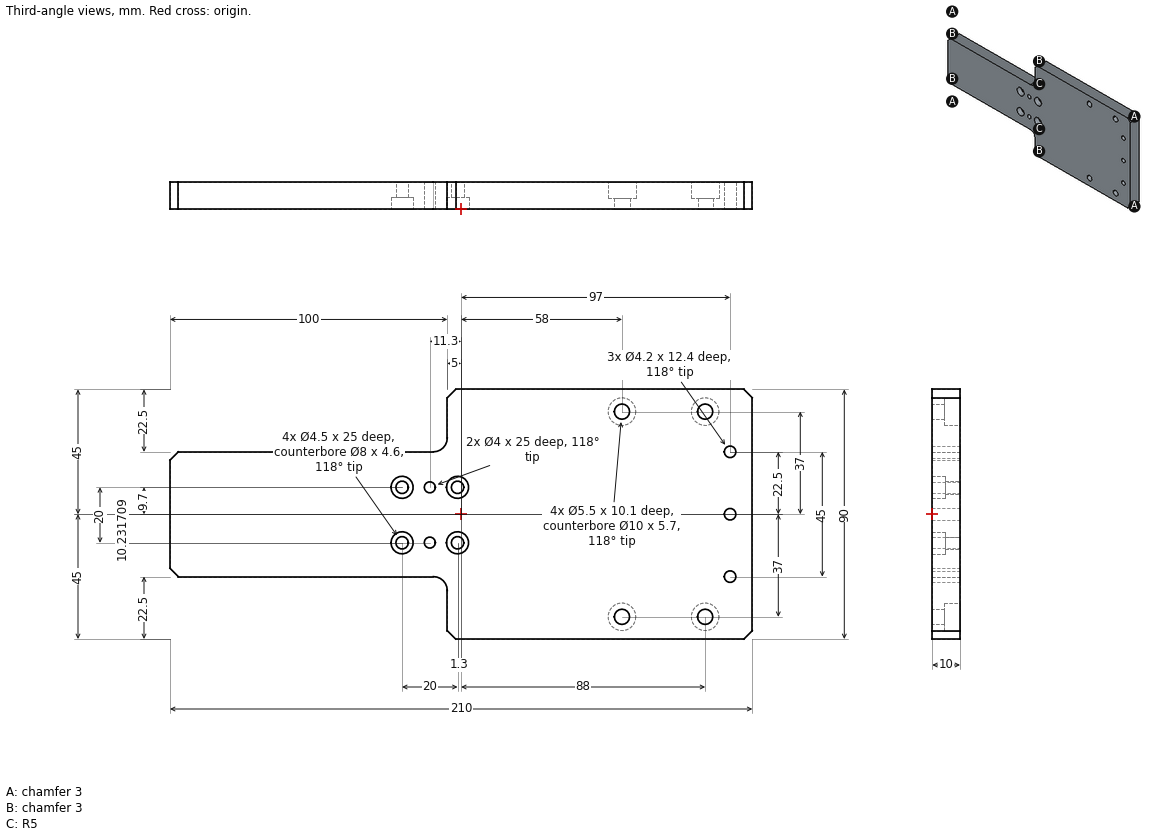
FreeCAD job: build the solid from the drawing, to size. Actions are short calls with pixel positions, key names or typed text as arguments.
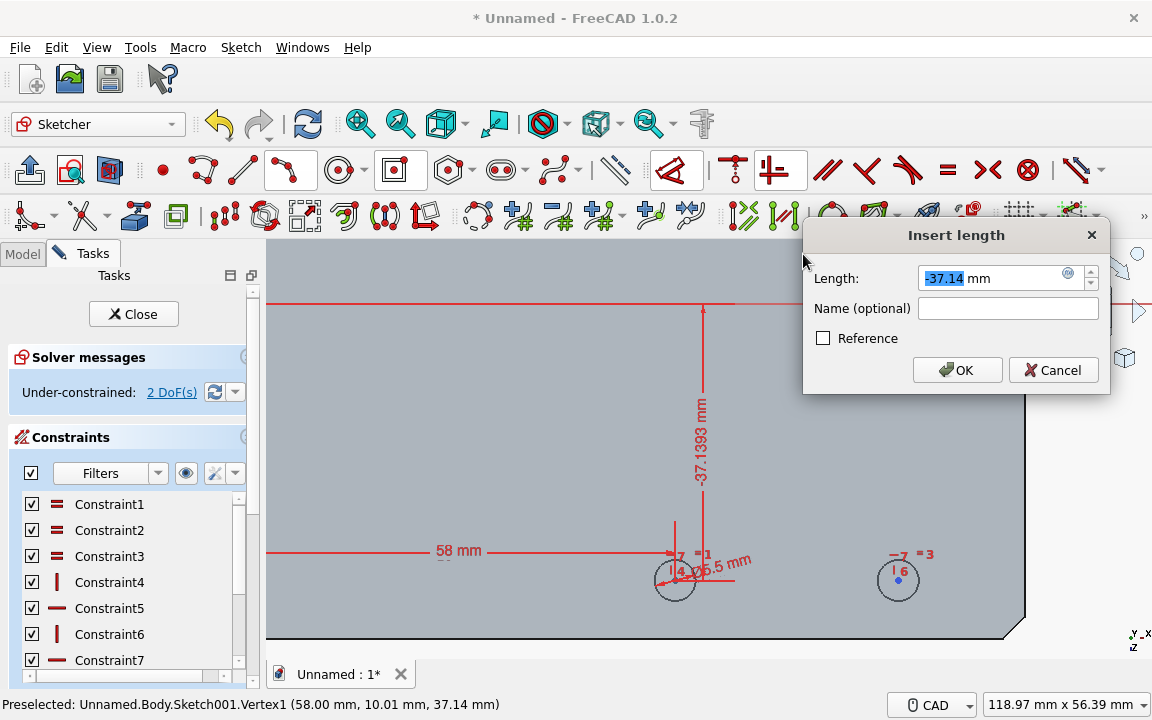
text(-37)
key(Return)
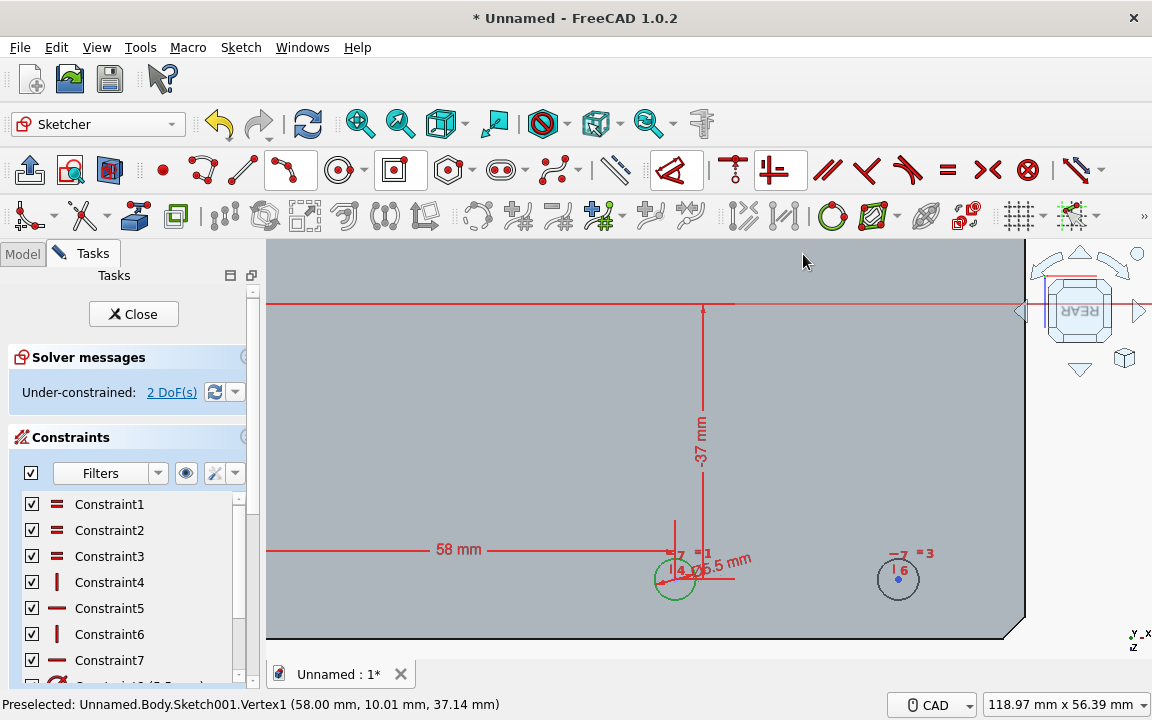
scroll(689, 567, down, 4)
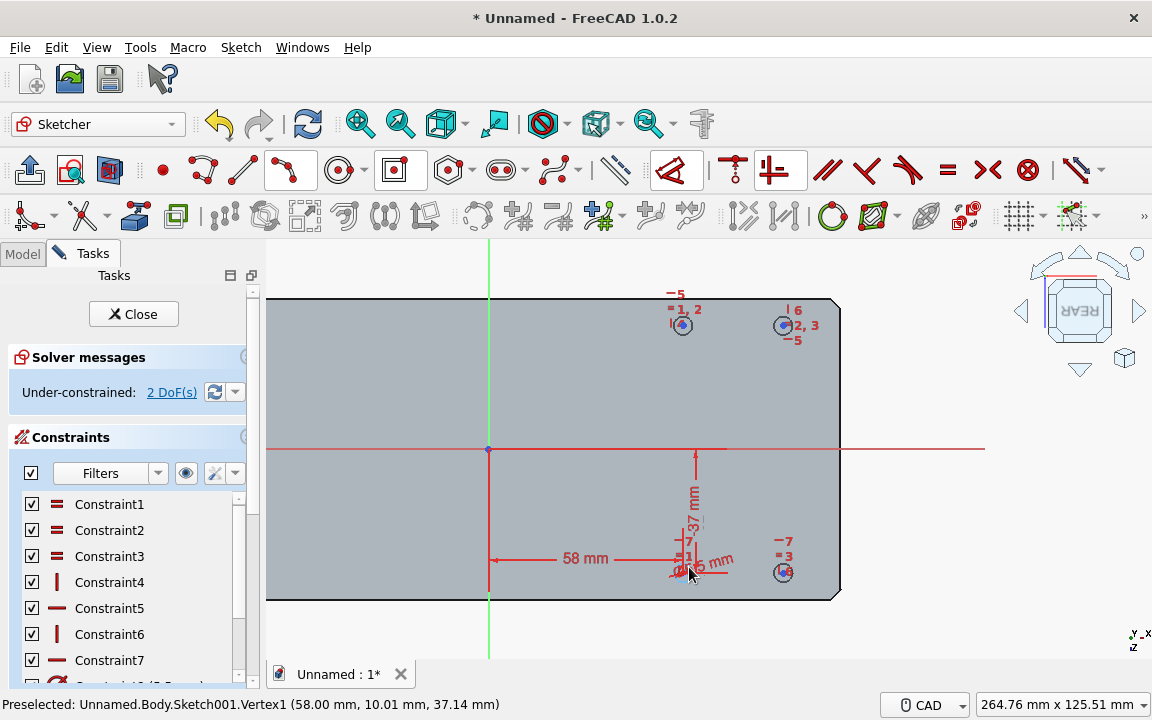
click(683, 326)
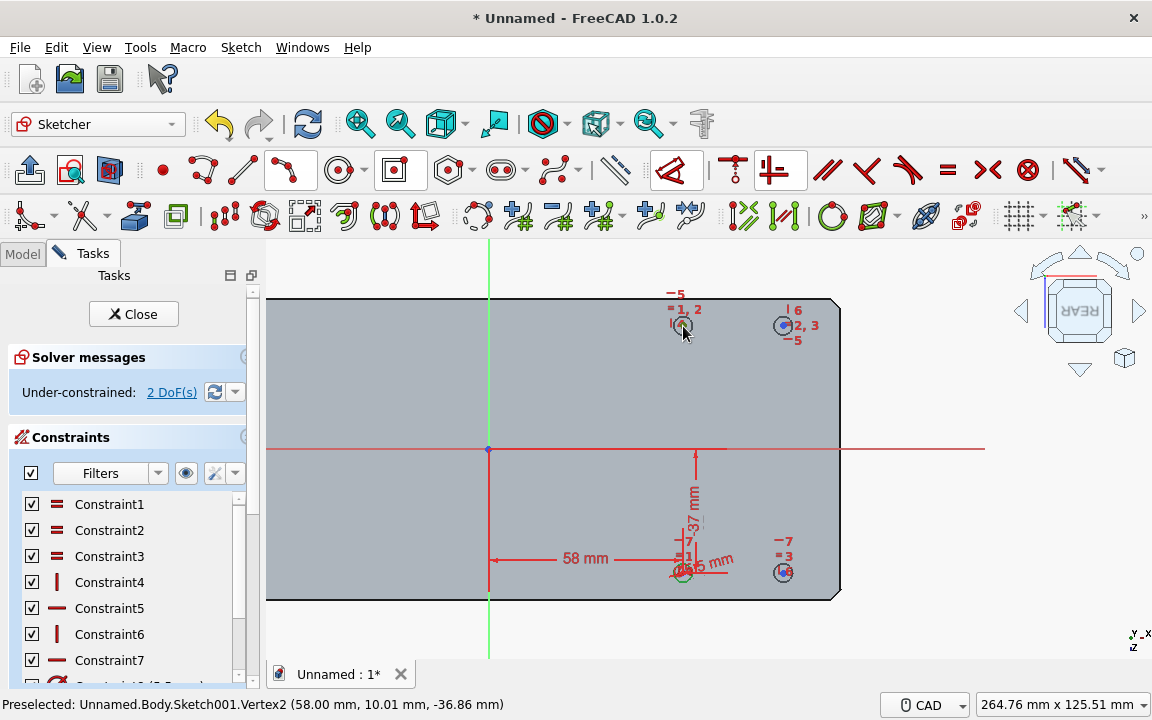
click(698, 170)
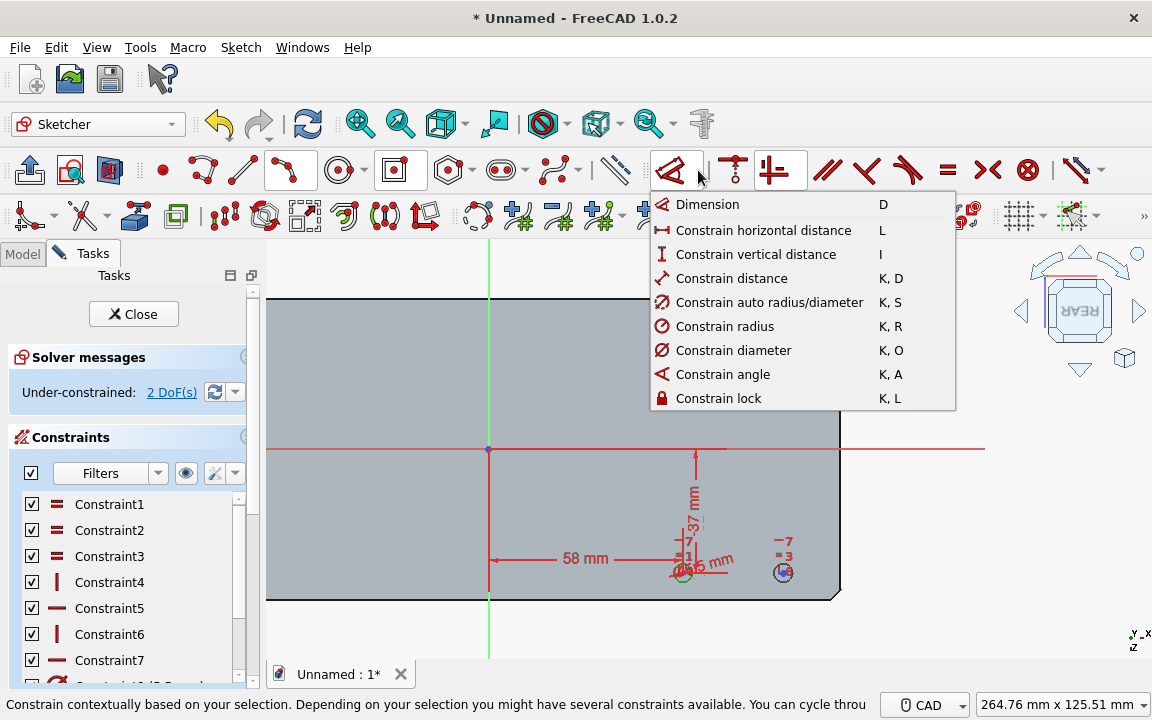
click(803, 254)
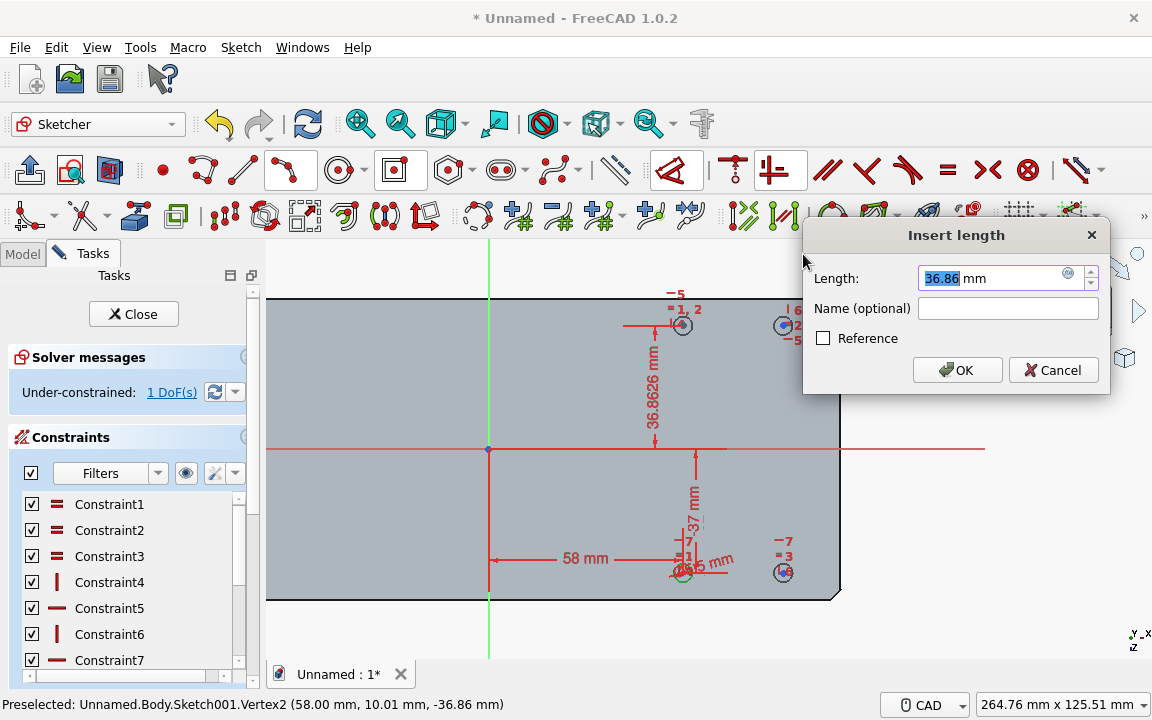
text(37)
key(Return)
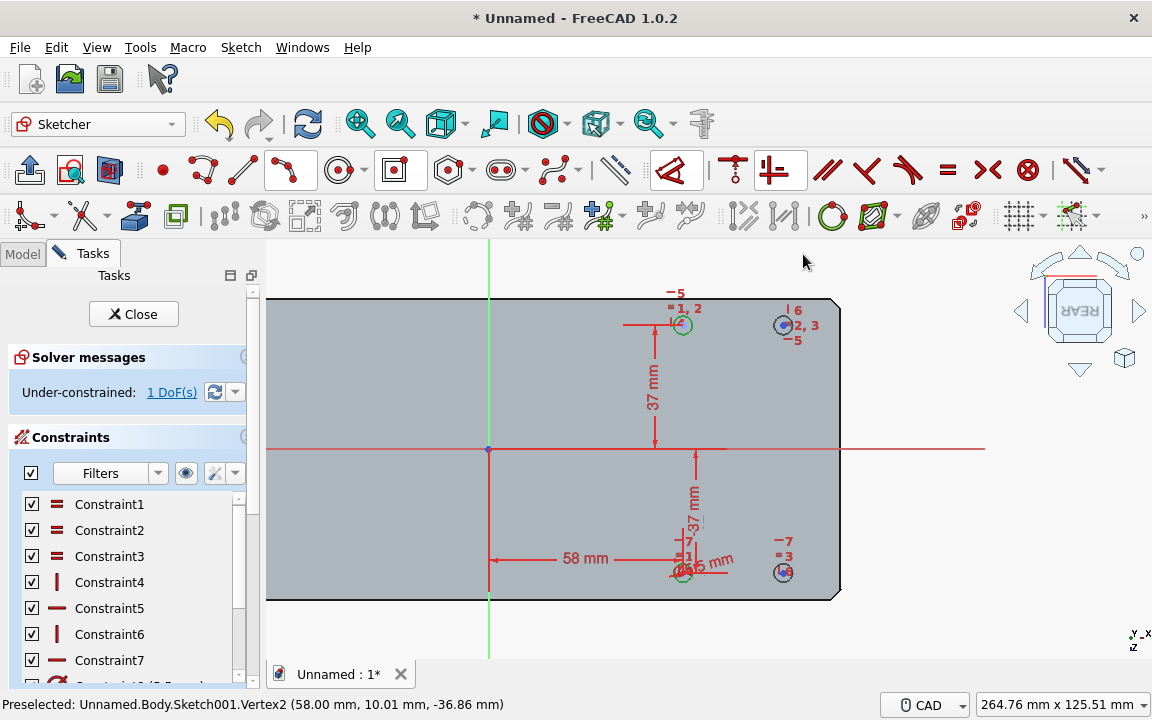
click(783, 325)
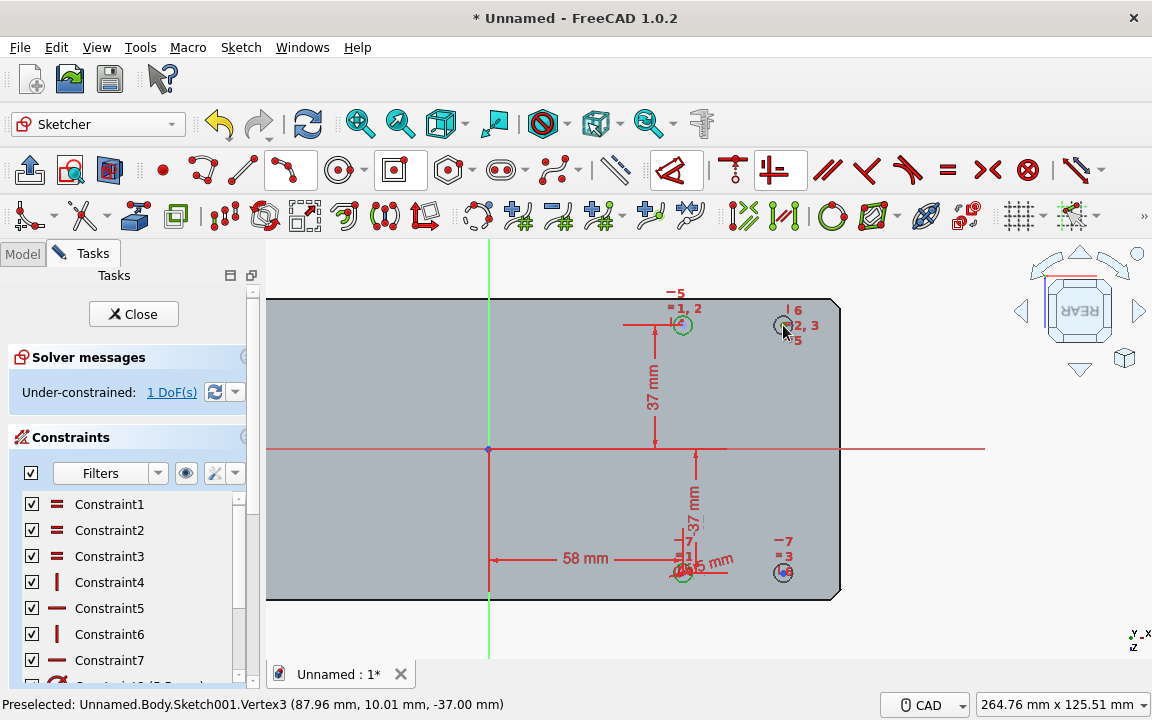
click(698, 170)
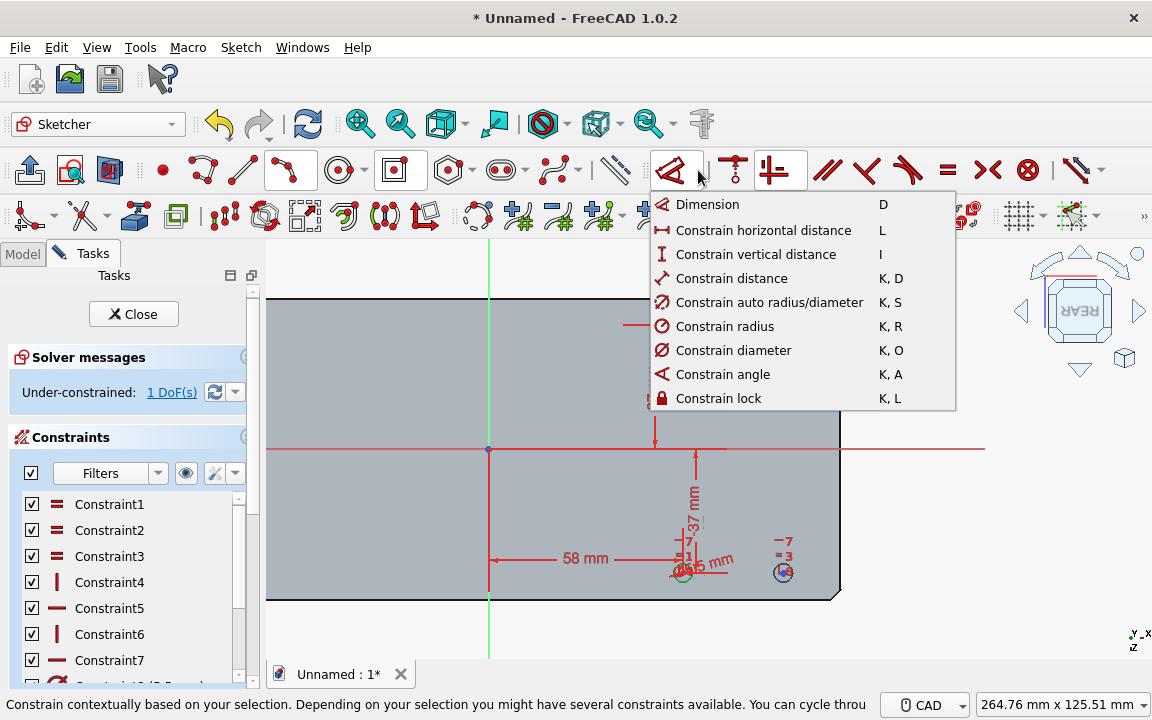
click(803, 230)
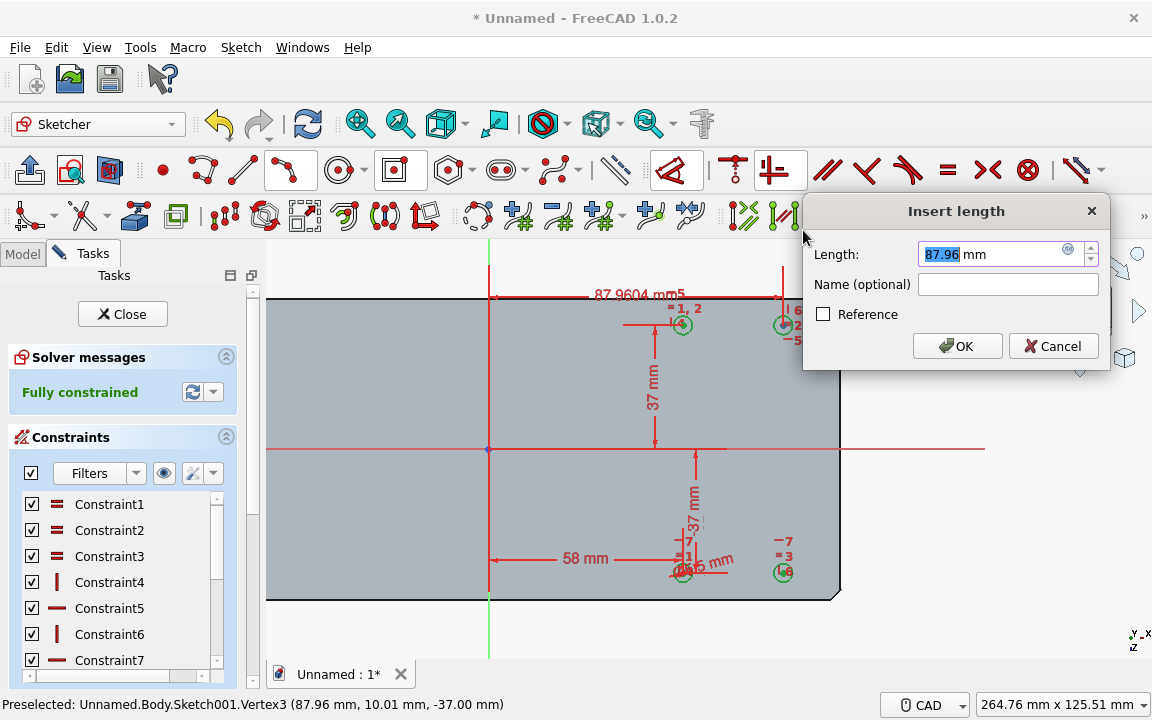
text(88)
key(Return)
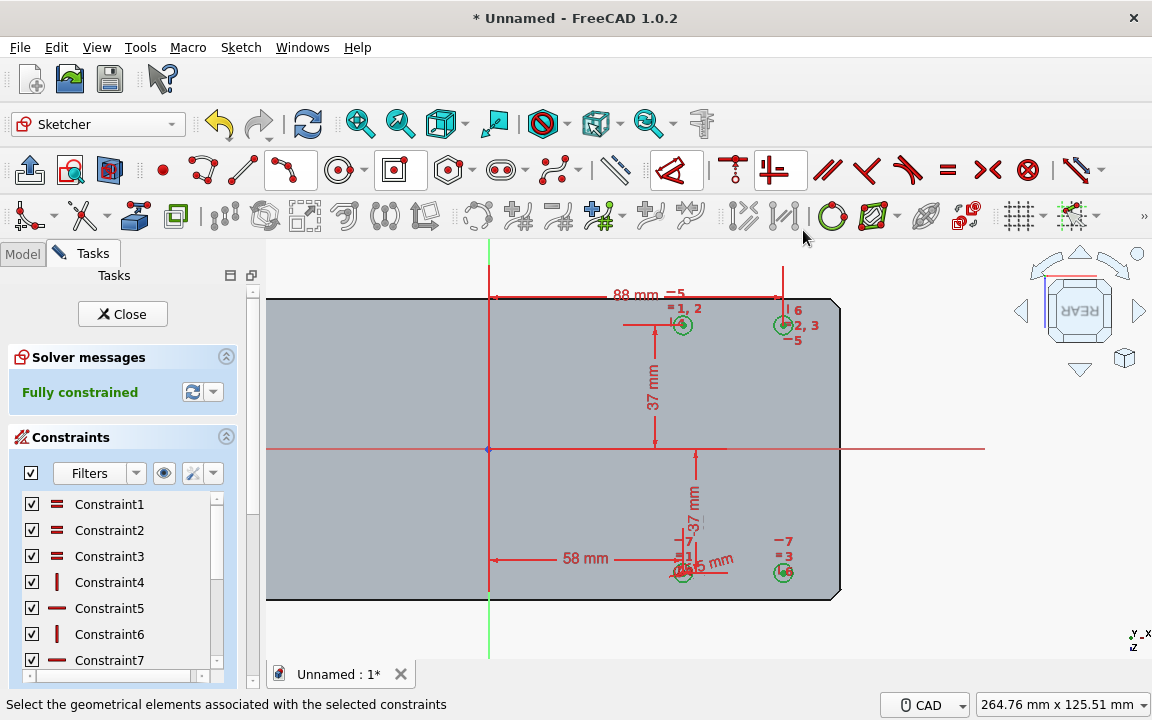
click(123, 314)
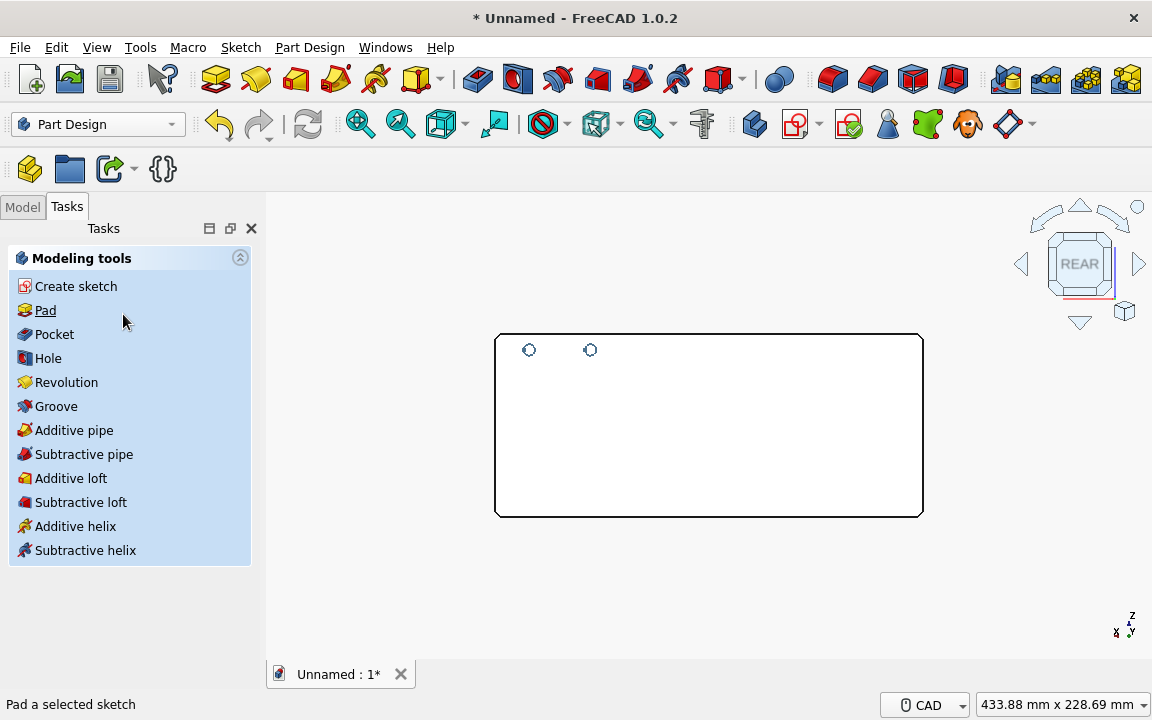
click(518, 80)